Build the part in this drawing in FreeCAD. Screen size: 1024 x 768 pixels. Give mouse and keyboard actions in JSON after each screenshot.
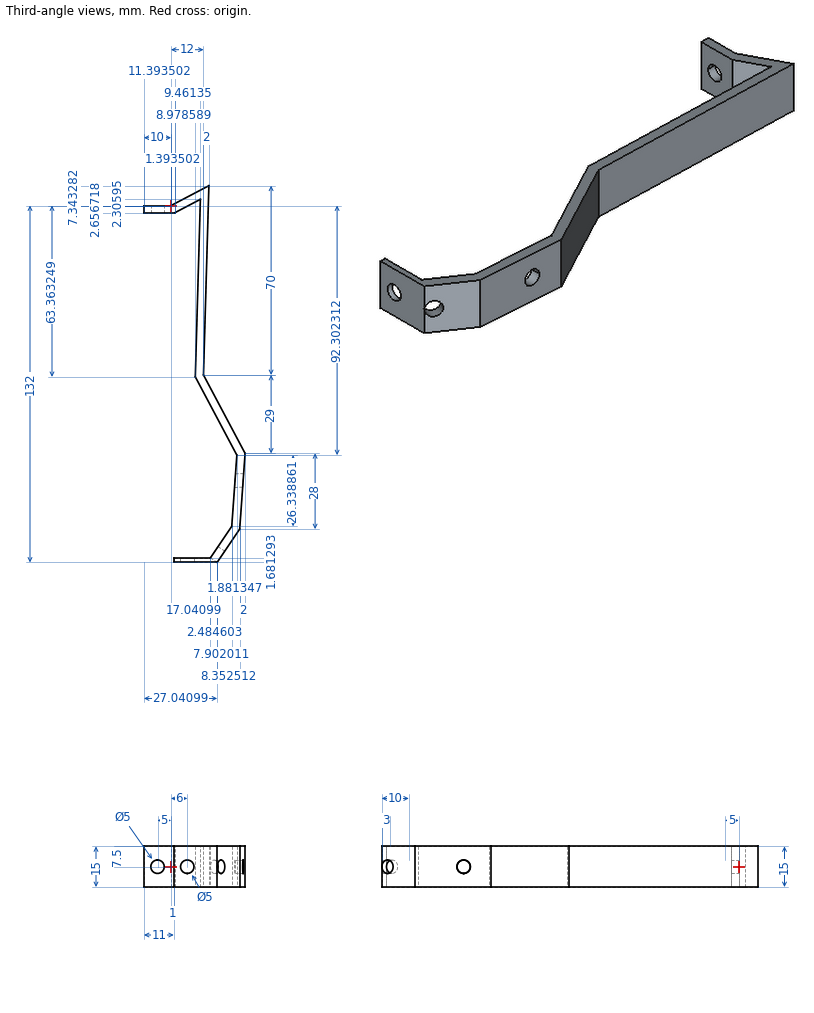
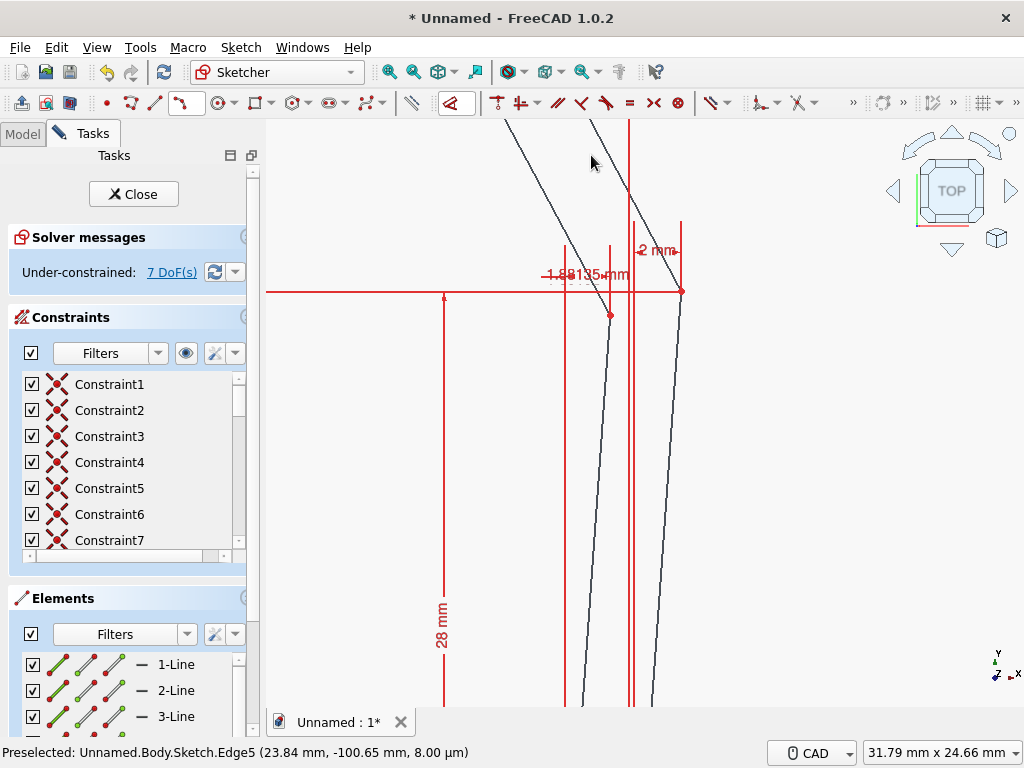
{"action": "scroll", "coordinate": [604, 515], "scroll_direction": "down", "scroll_amount": 11}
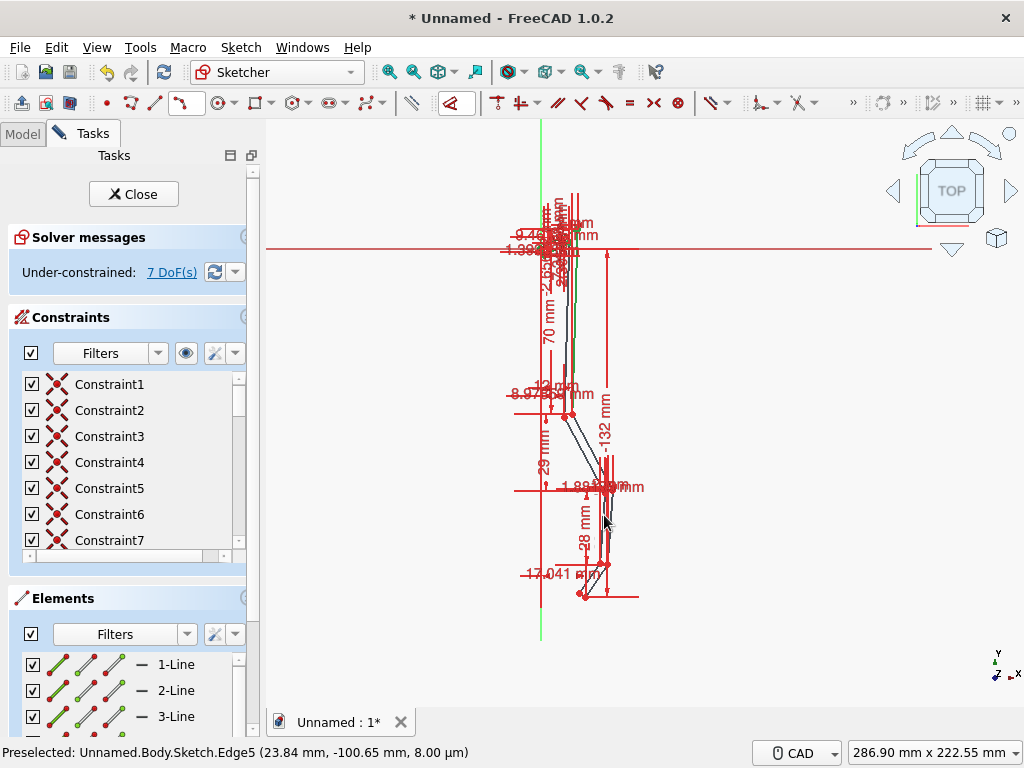
{"action": "scroll", "coordinate": [594, 573], "scroll_direction": "up", "scroll_amount": 4}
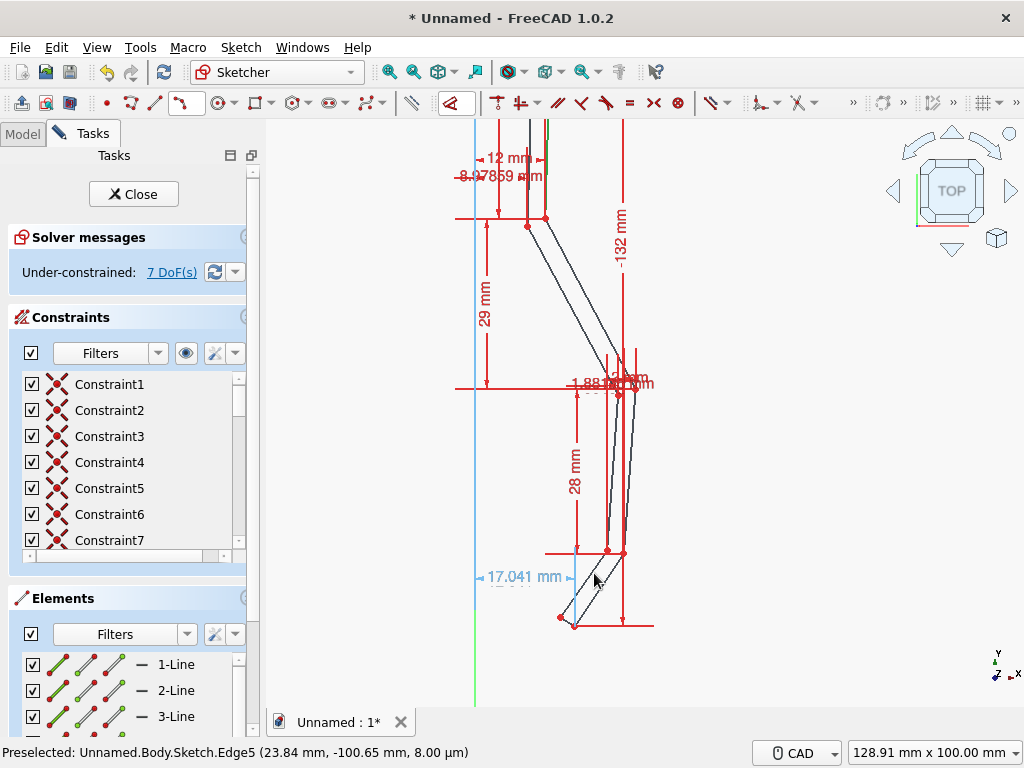
{"action": "left_click", "coordinate": [593, 571]}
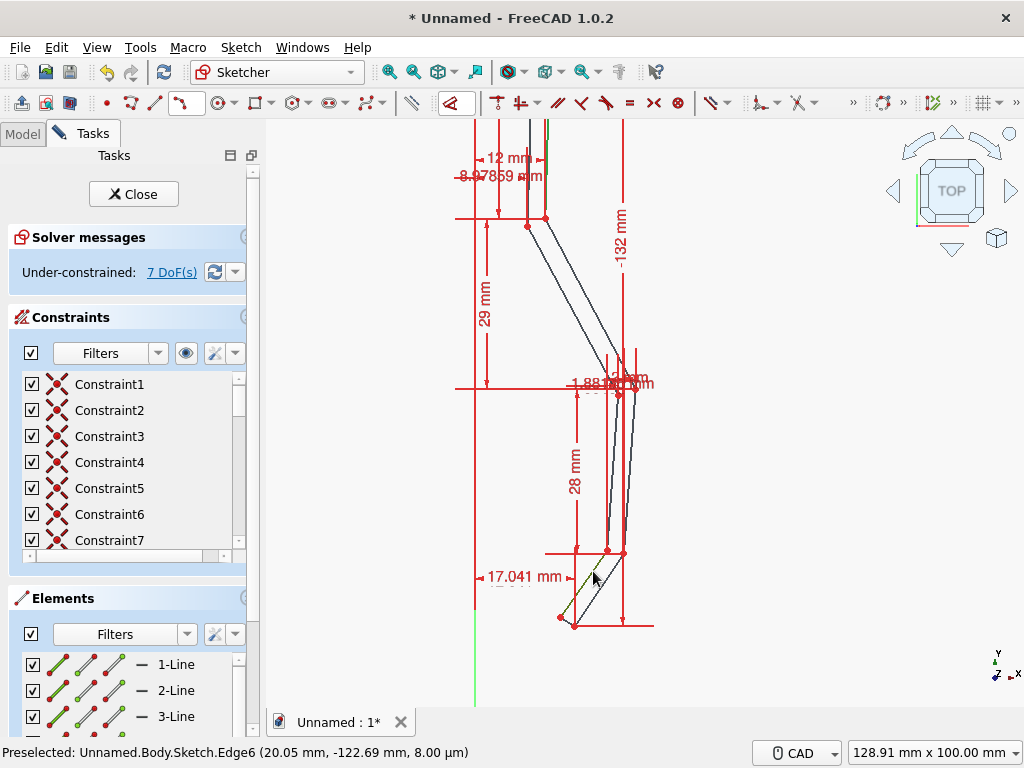
{"action": "key", "text": "l"}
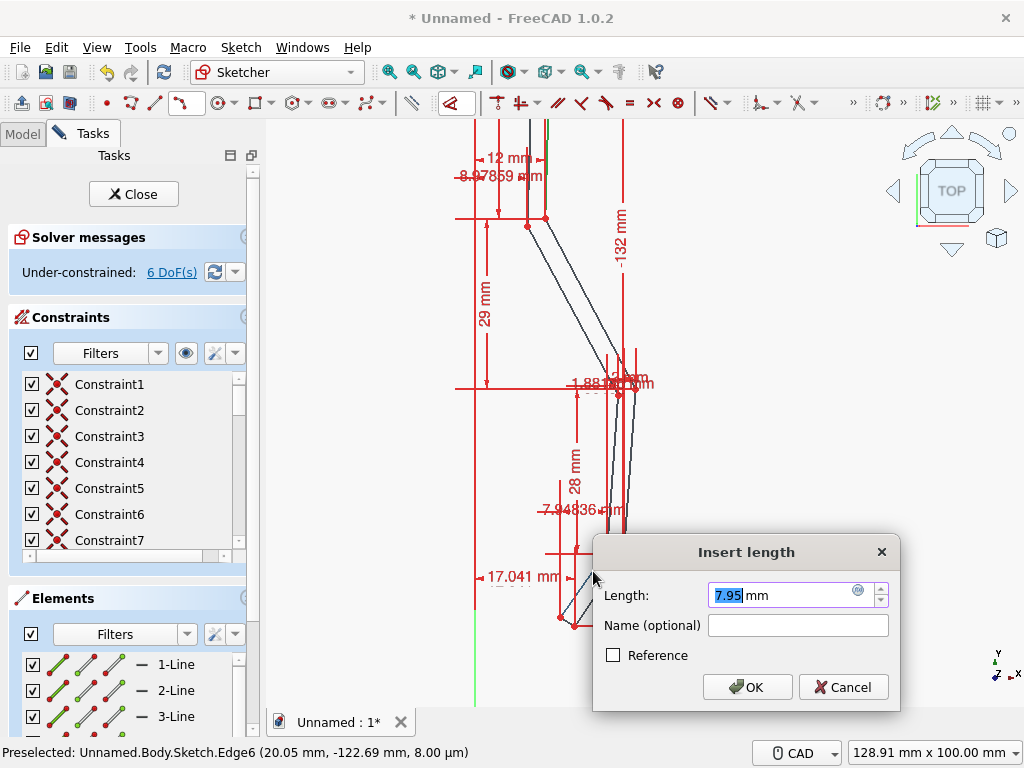
{"action": "type", "text": "7.902011"}
{"action": "key", "text": "Return"}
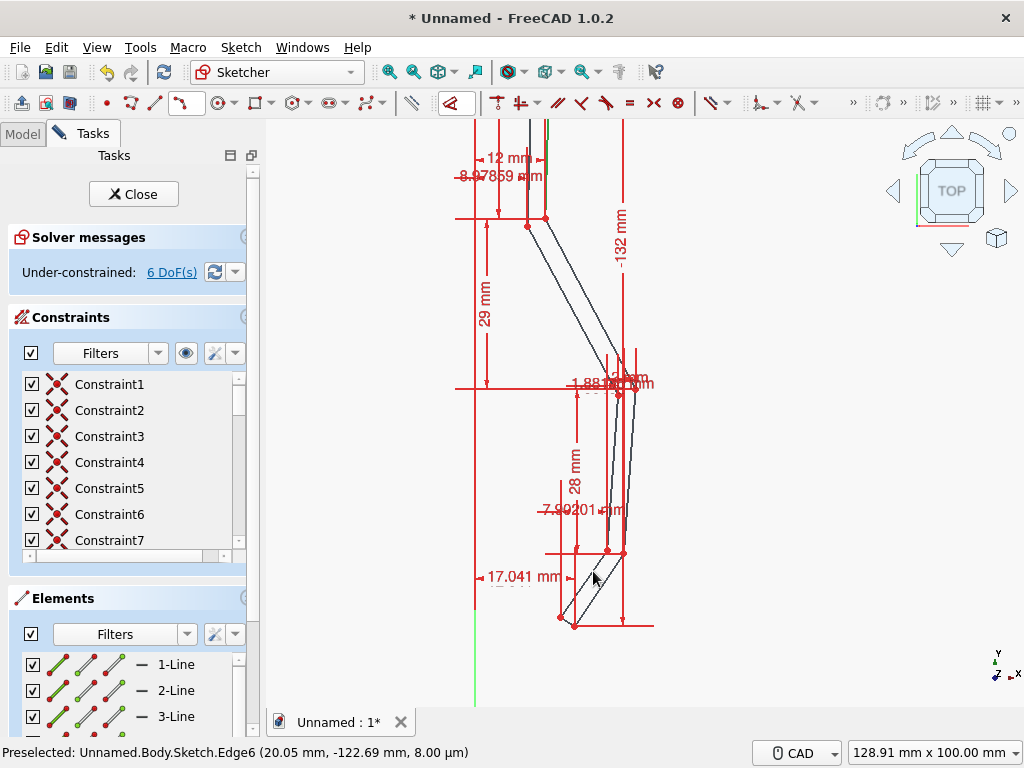
{"action": "scroll", "coordinate": [568, 622], "scroll_direction": "up", "scroll_amount": 5}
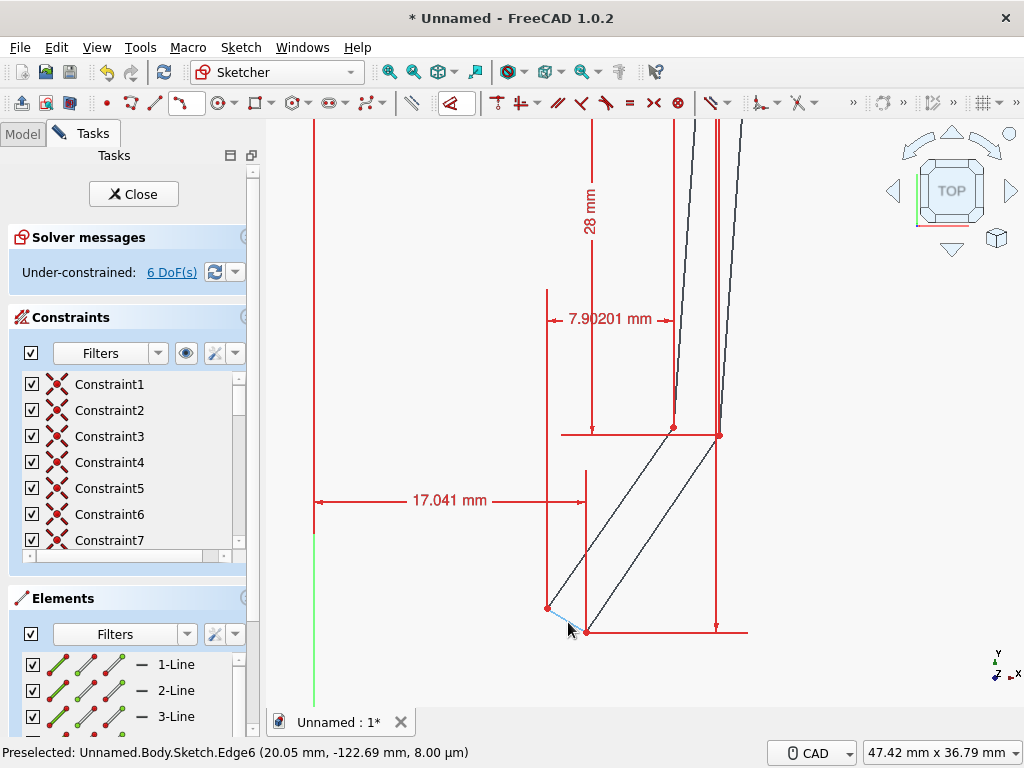
{"action": "left_click", "coordinate": [567, 621]}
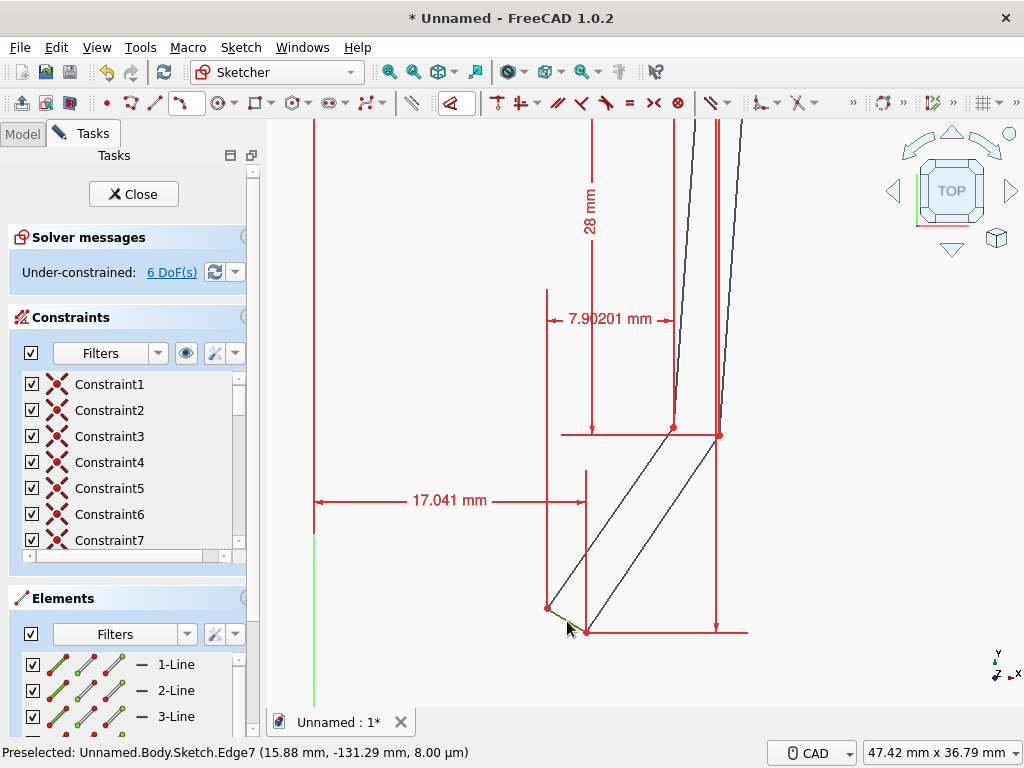
{"action": "key", "text": "l"}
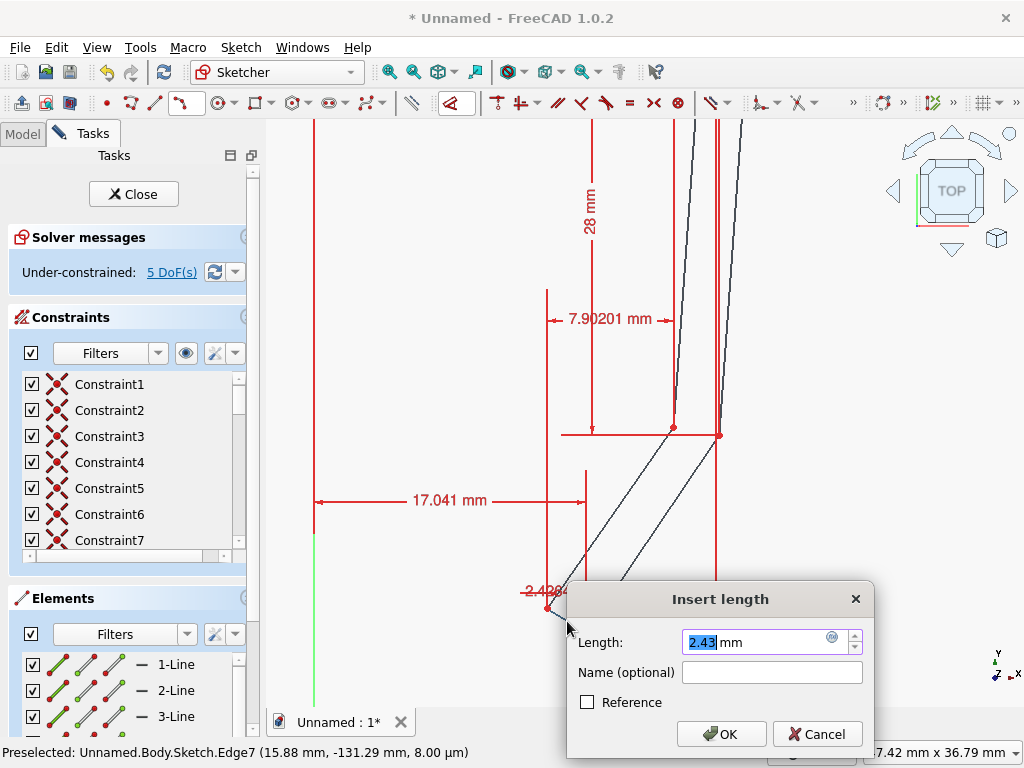
{"action": "type", "text": "2.484603"}
{"action": "key", "text": "Return"}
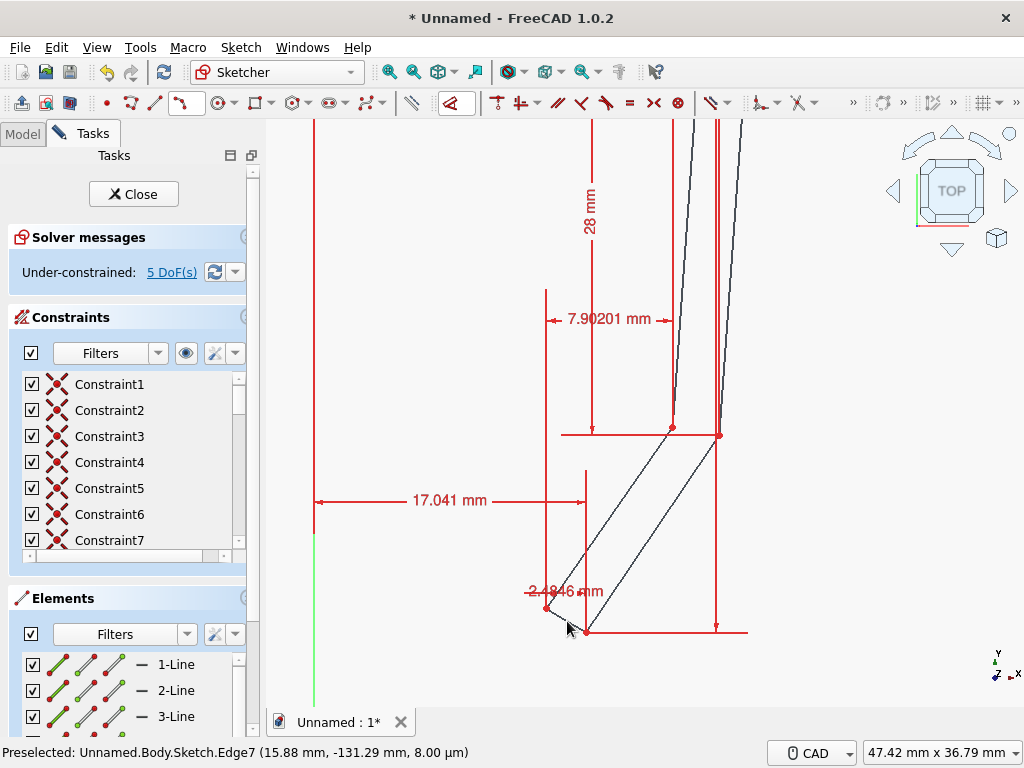
{"action": "scroll", "coordinate": [558, 616], "scroll_direction": "up", "scroll_amount": 2}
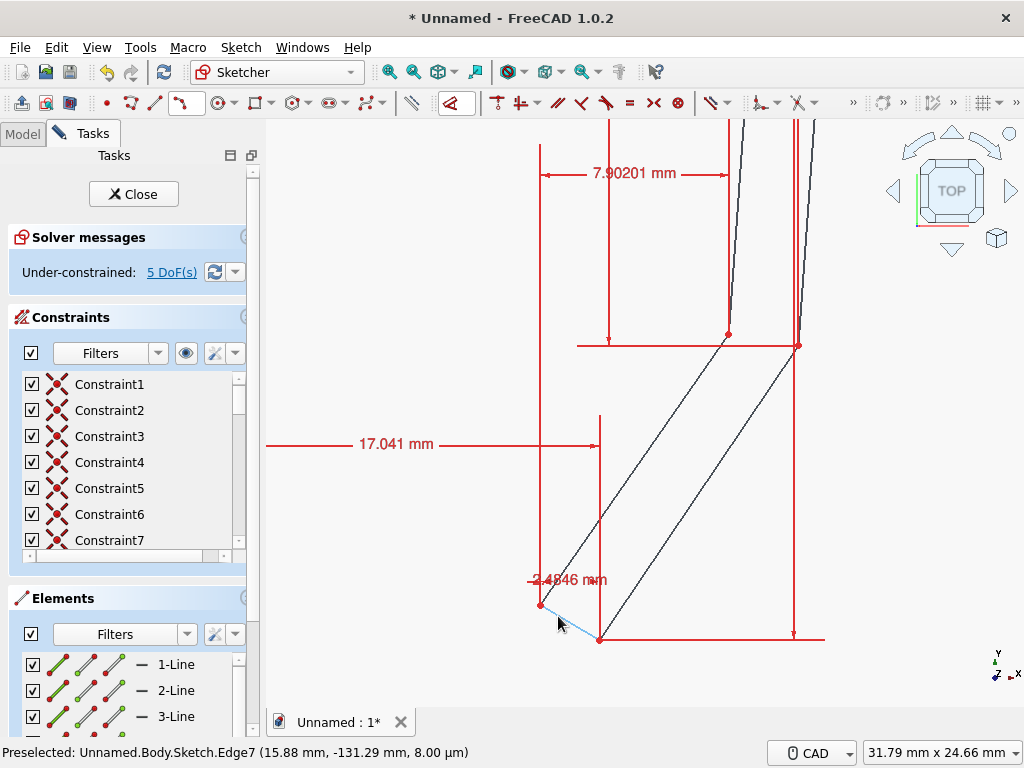
{"action": "left_click", "coordinate": [558, 616]}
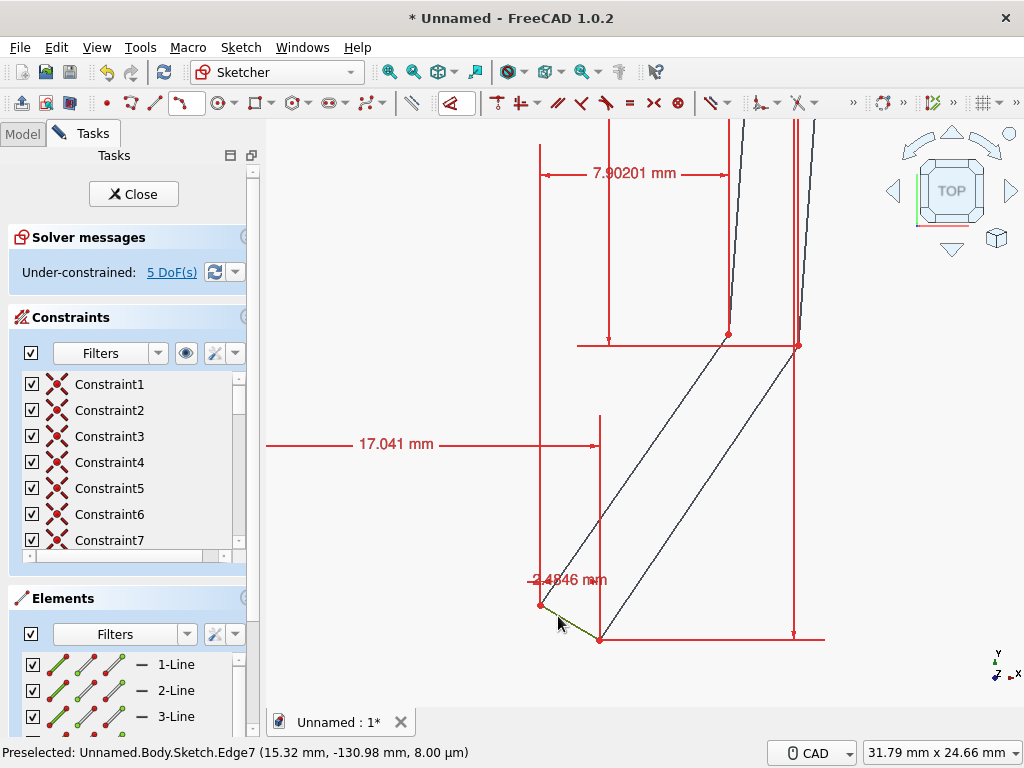
{"action": "left_click", "coordinate": [470, 104]}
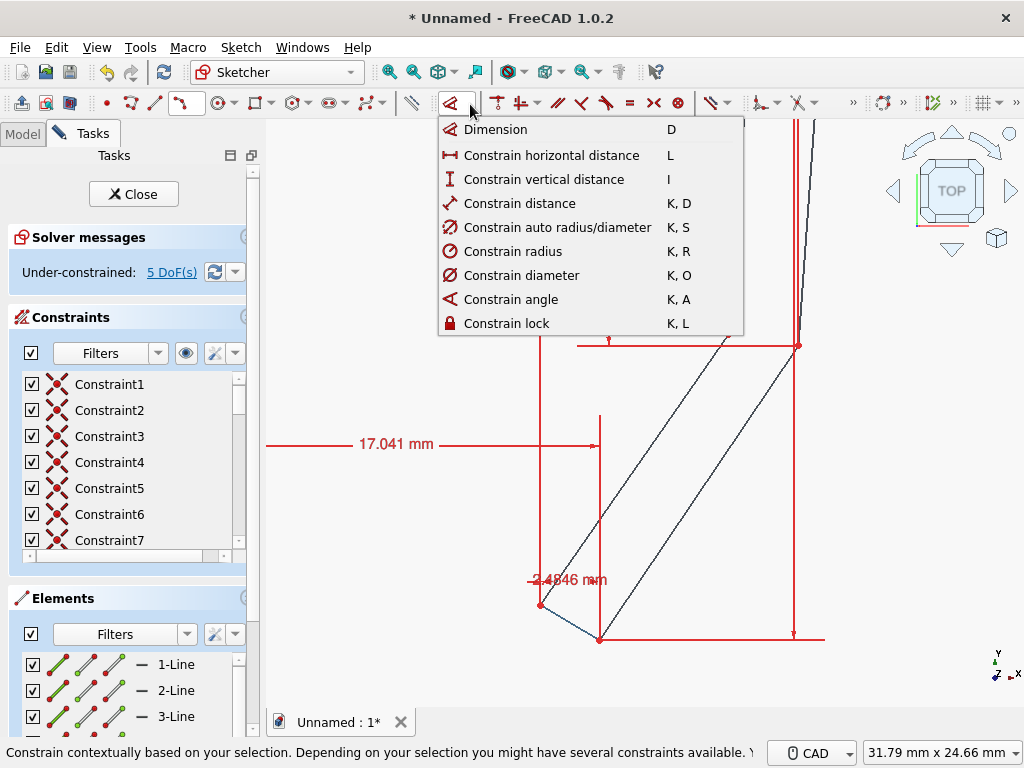
{"action": "left_click", "coordinate": [591, 179]}